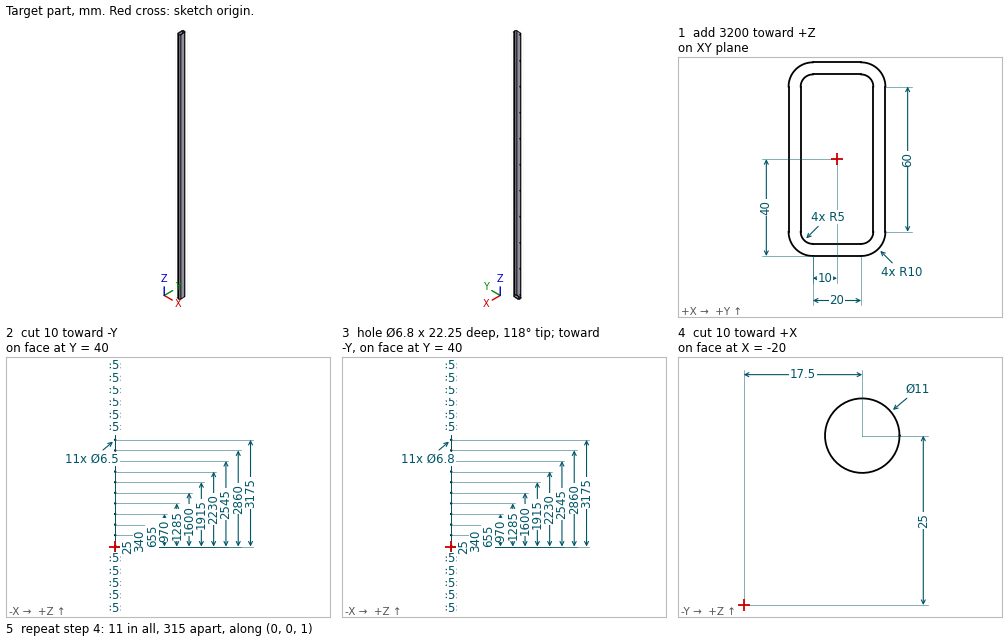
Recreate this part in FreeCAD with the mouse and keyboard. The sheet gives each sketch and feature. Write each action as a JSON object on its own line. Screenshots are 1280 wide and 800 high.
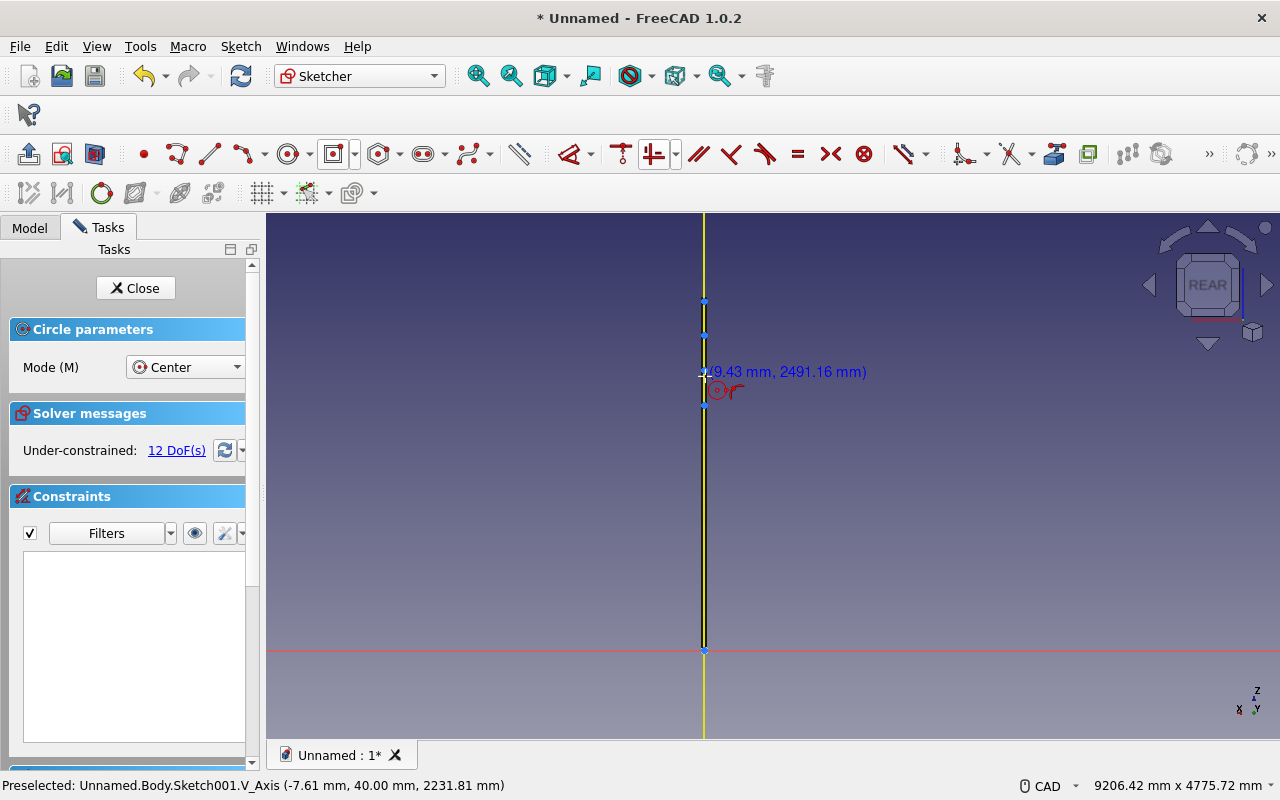
{"action": "scroll", "coordinate": [705, 440], "scroll_direction": "up", "scroll_amount": 21}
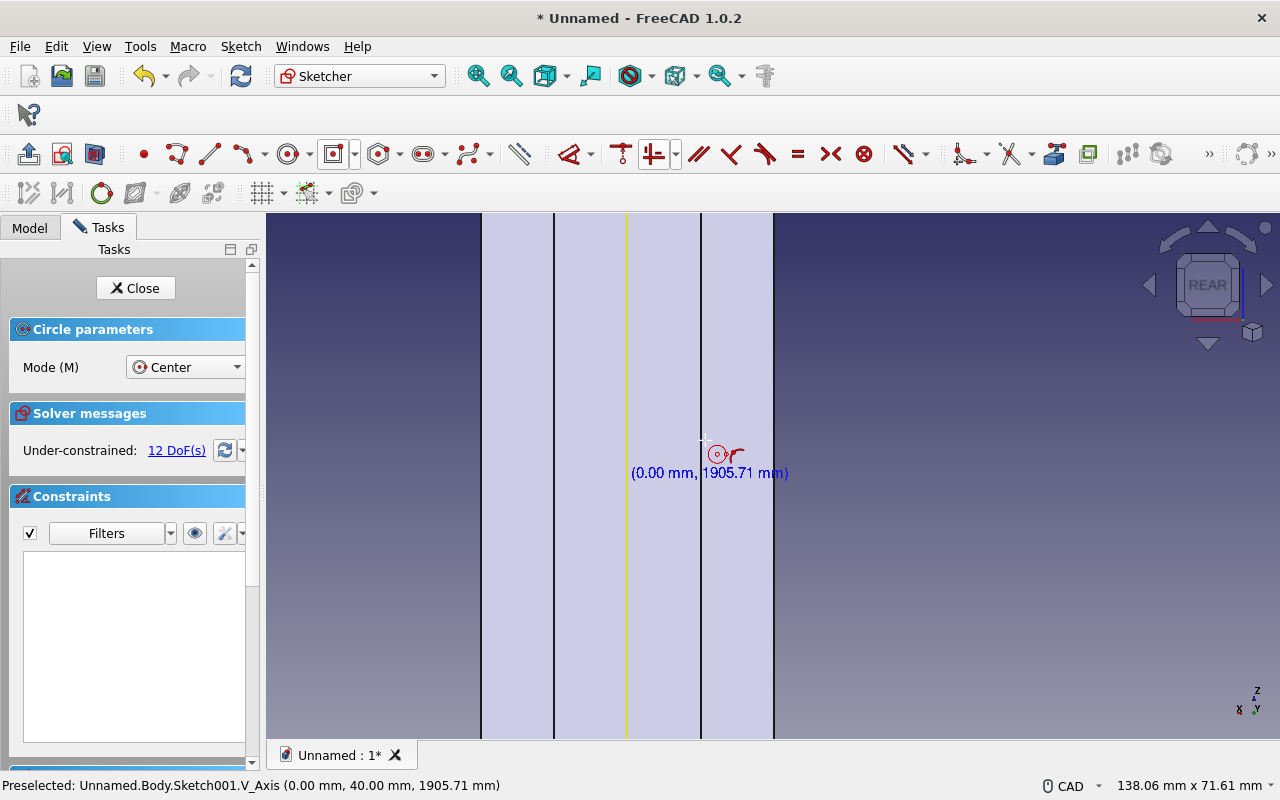
{"action": "left_click", "coordinate": [664, 410]}
{"action": "left_click", "coordinate": [681, 393]}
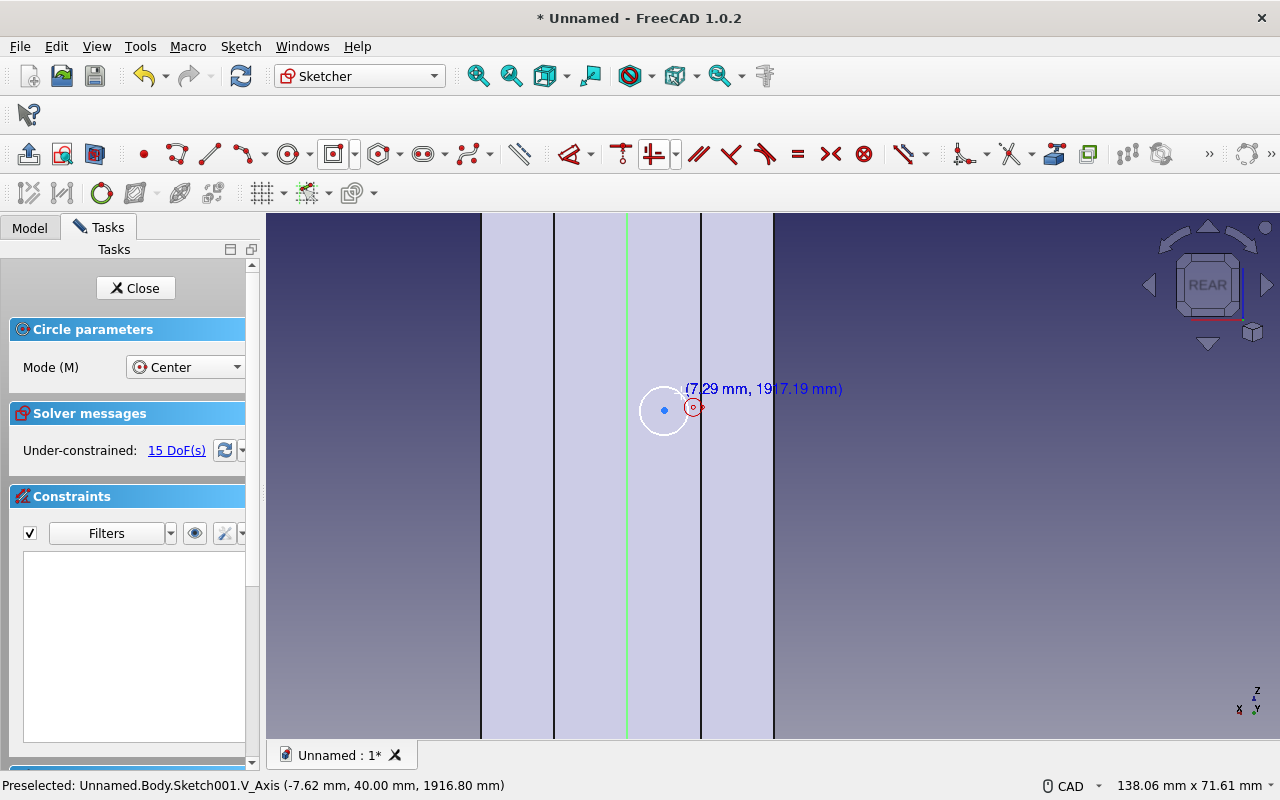
{"action": "scroll", "coordinate": [704, 476], "scroll_direction": "down", "scroll_amount": 15}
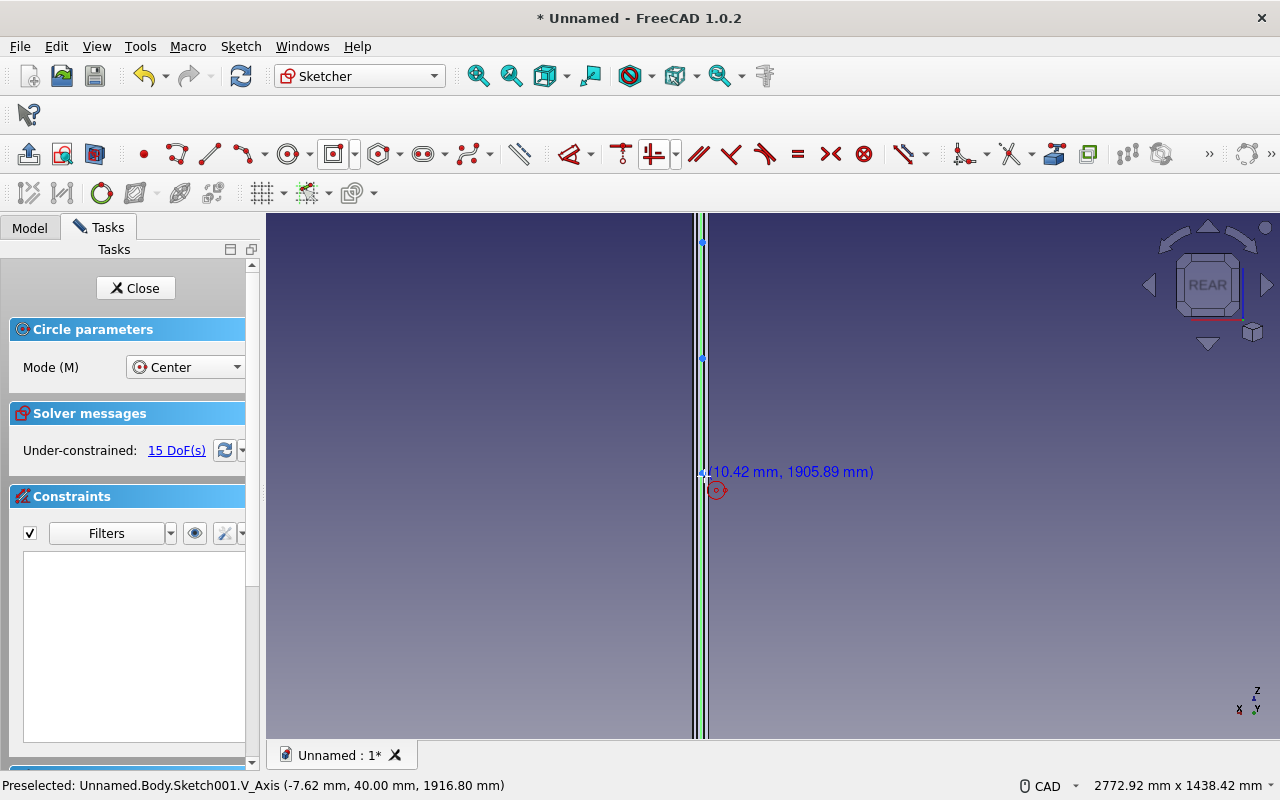
{"action": "scroll", "coordinate": [706, 426], "scroll_direction": "down", "scroll_amount": 6}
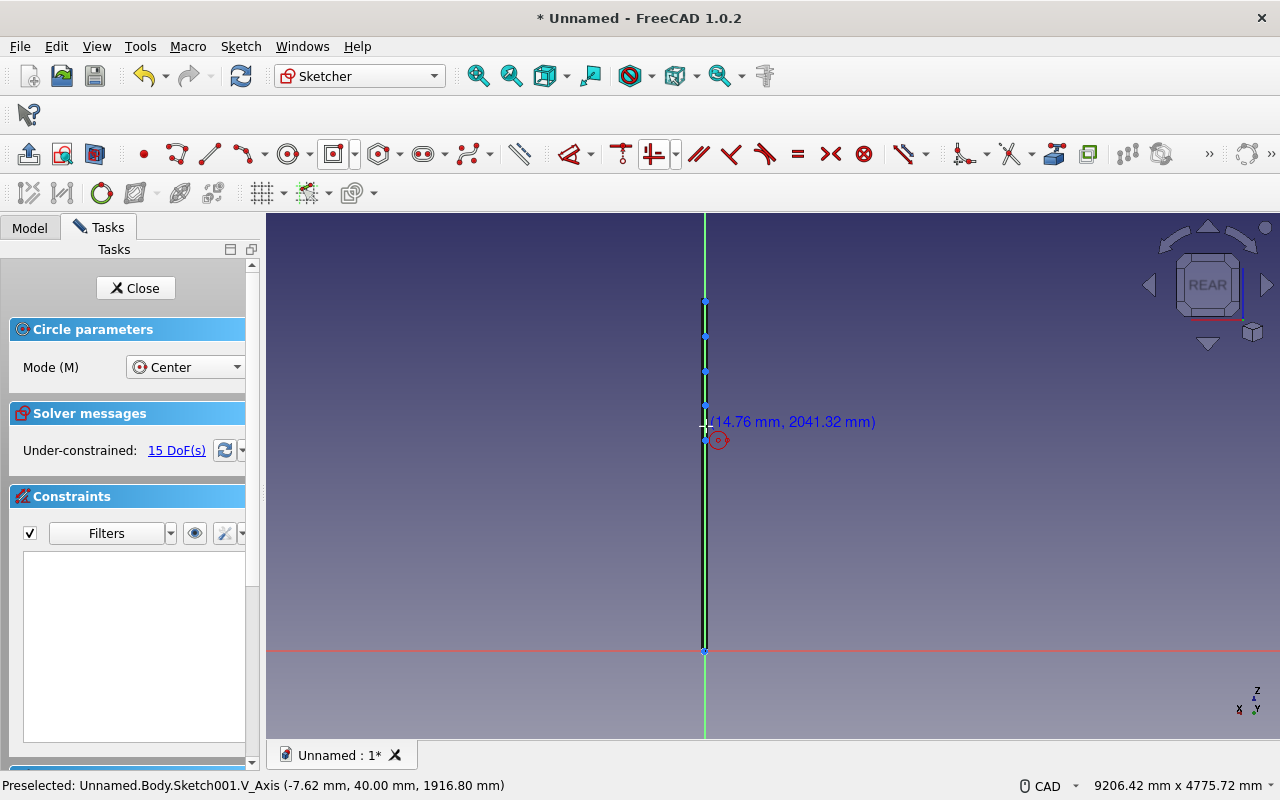
{"action": "scroll", "coordinate": [705, 475], "scroll_direction": "up", "scroll_amount": 21}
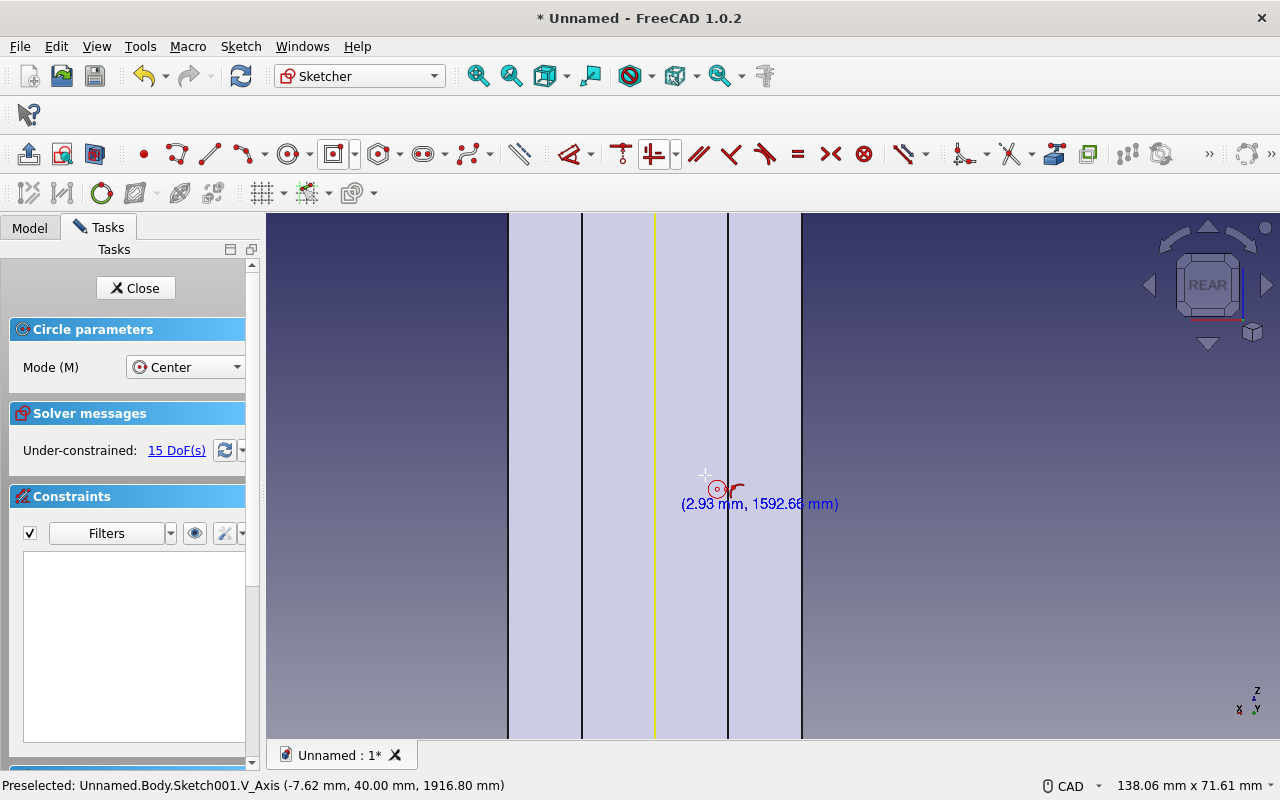
{"action": "left_click", "coordinate": [692, 455]}
{"action": "left_click", "coordinate": [709, 438]}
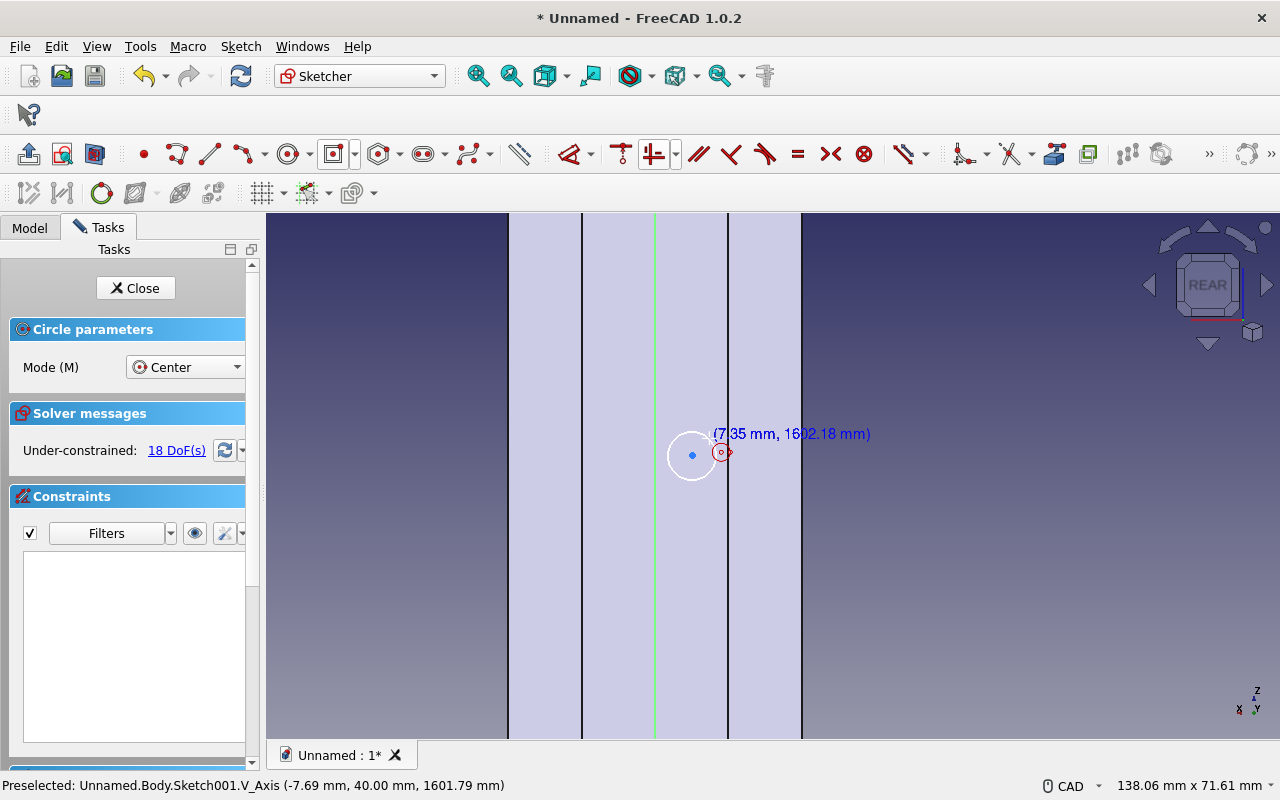
{"action": "scroll", "coordinate": [704, 476], "scroll_direction": "down", "scroll_amount": 15}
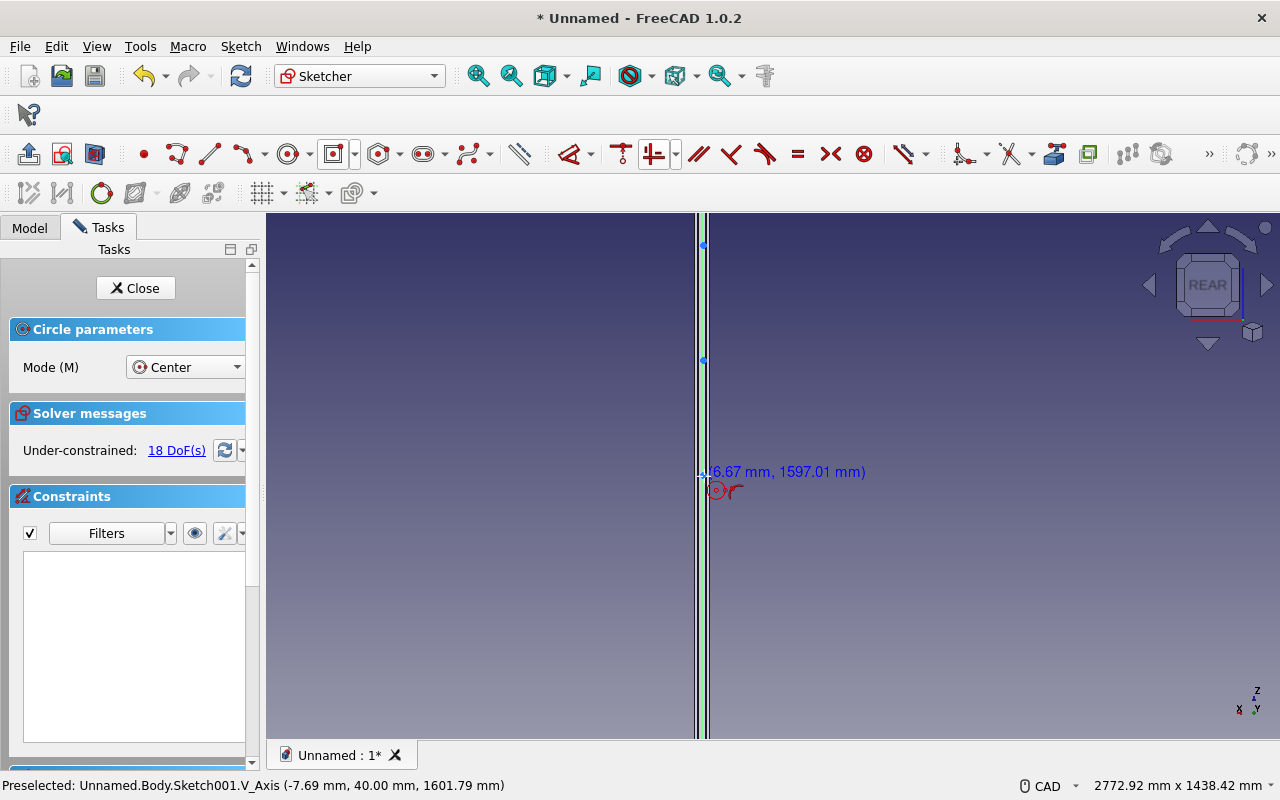
{"action": "scroll", "coordinate": [705, 475], "scroll_direction": "down", "scroll_amount": 6}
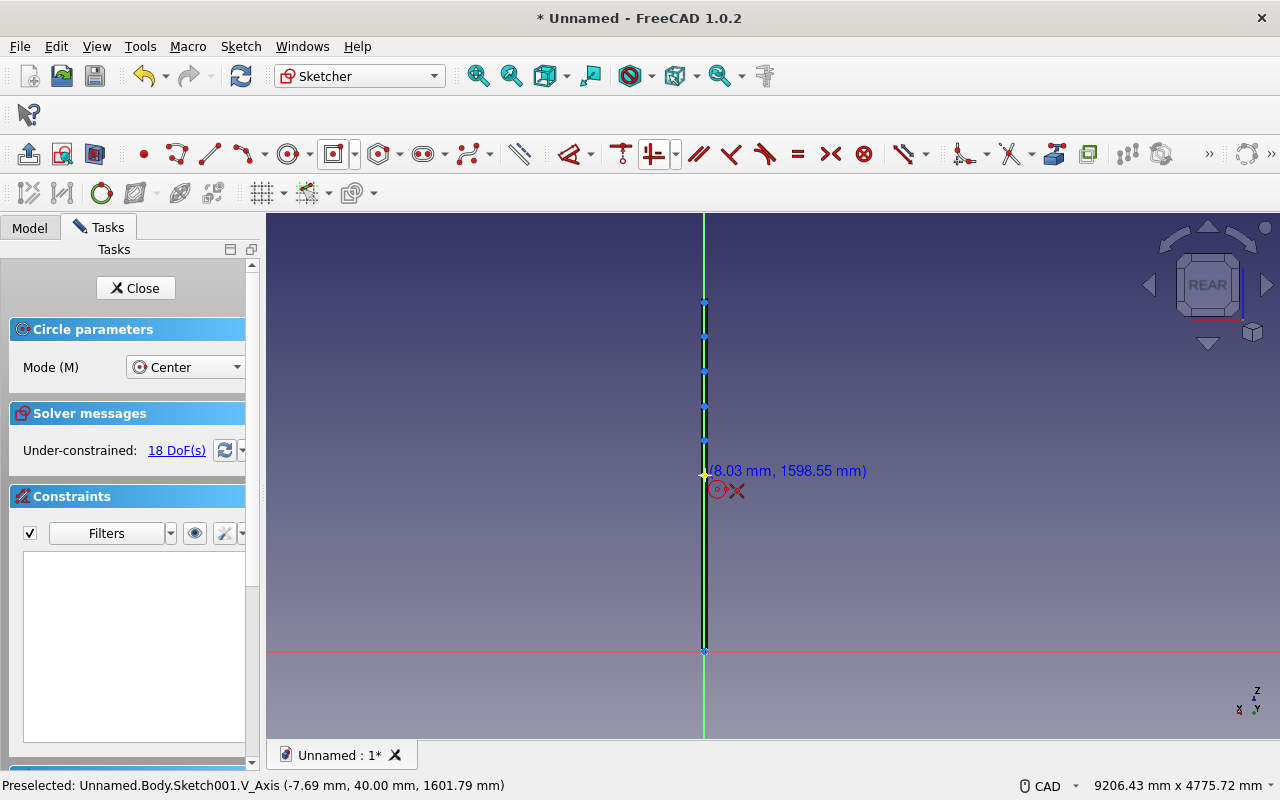
{"action": "scroll", "coordinate": [705, 510], "scroll_direction": "up", "scroll_amount": 21}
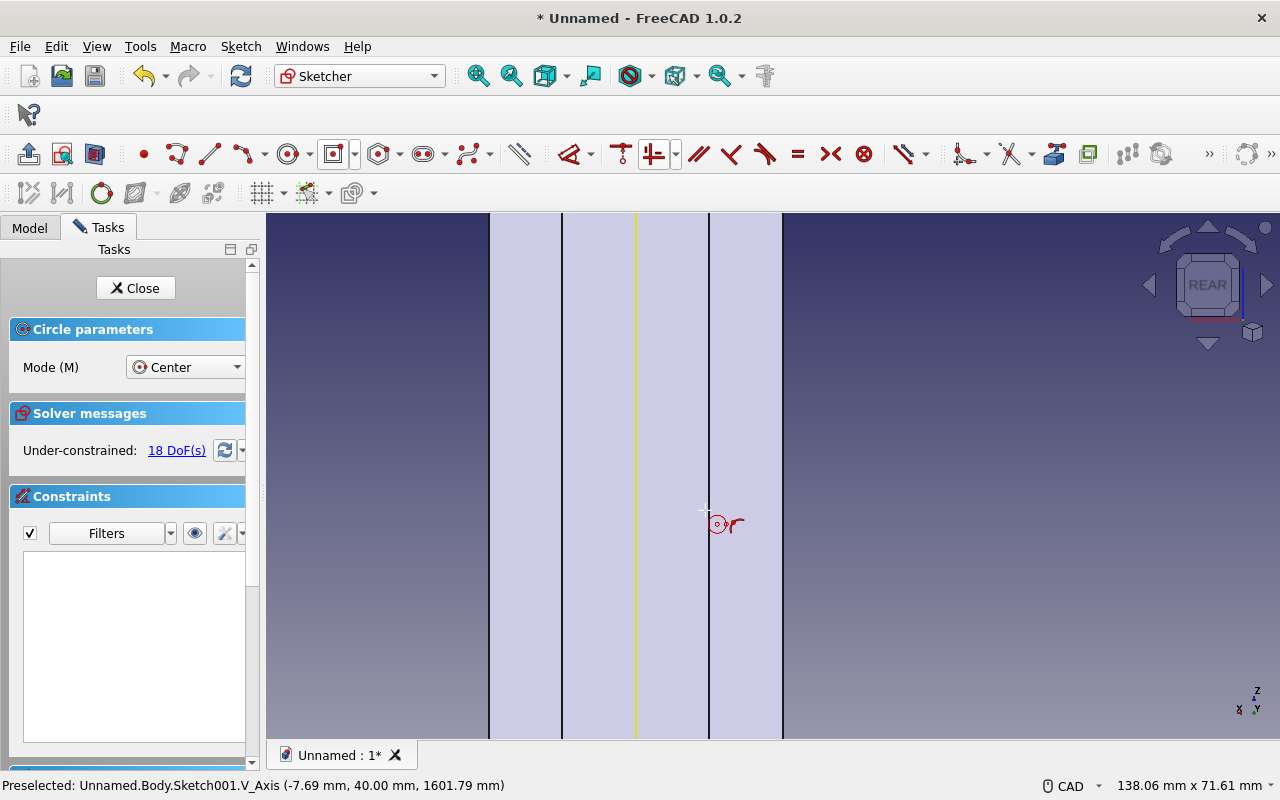
{"action": "left_click", "coordinate": [673, 484]}
{"action": "left_click", "coordinate": [690, 467]}